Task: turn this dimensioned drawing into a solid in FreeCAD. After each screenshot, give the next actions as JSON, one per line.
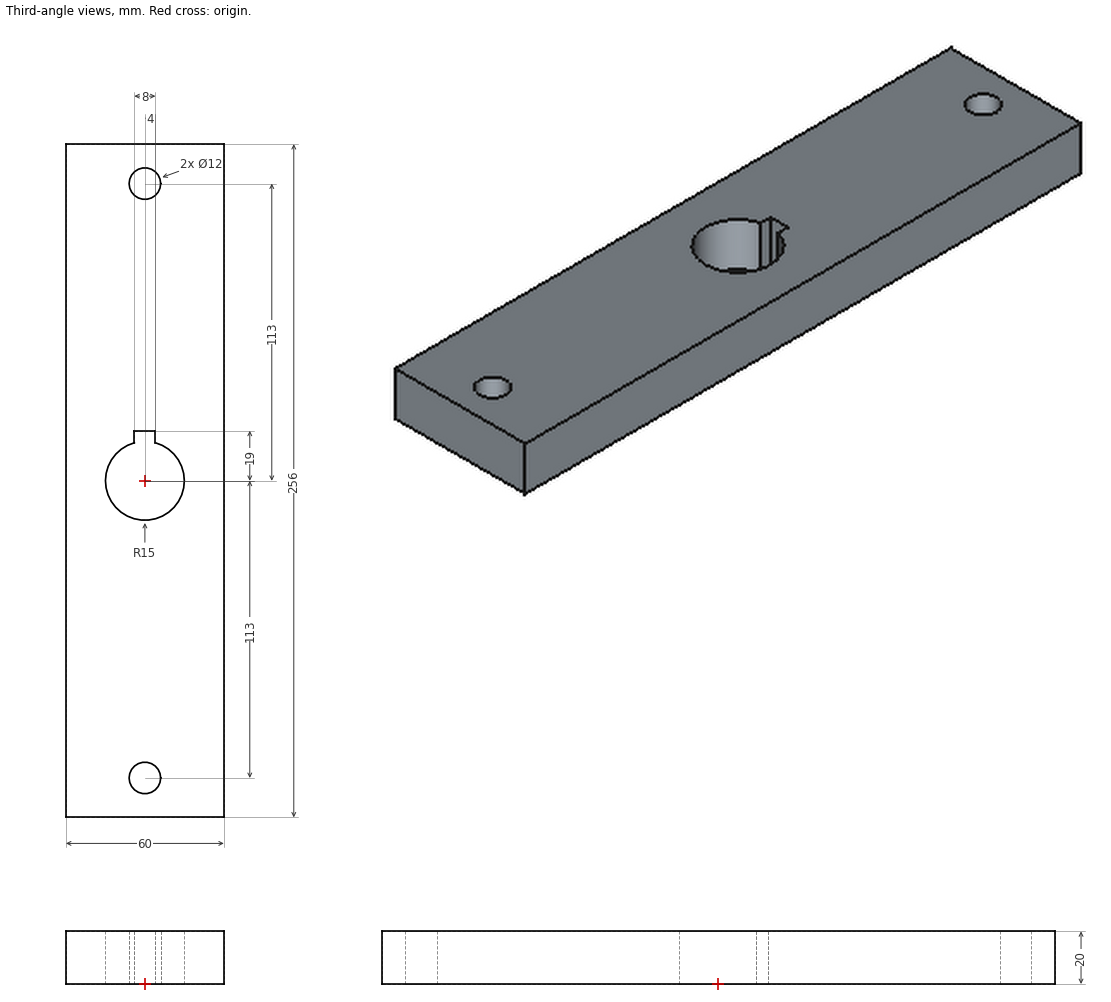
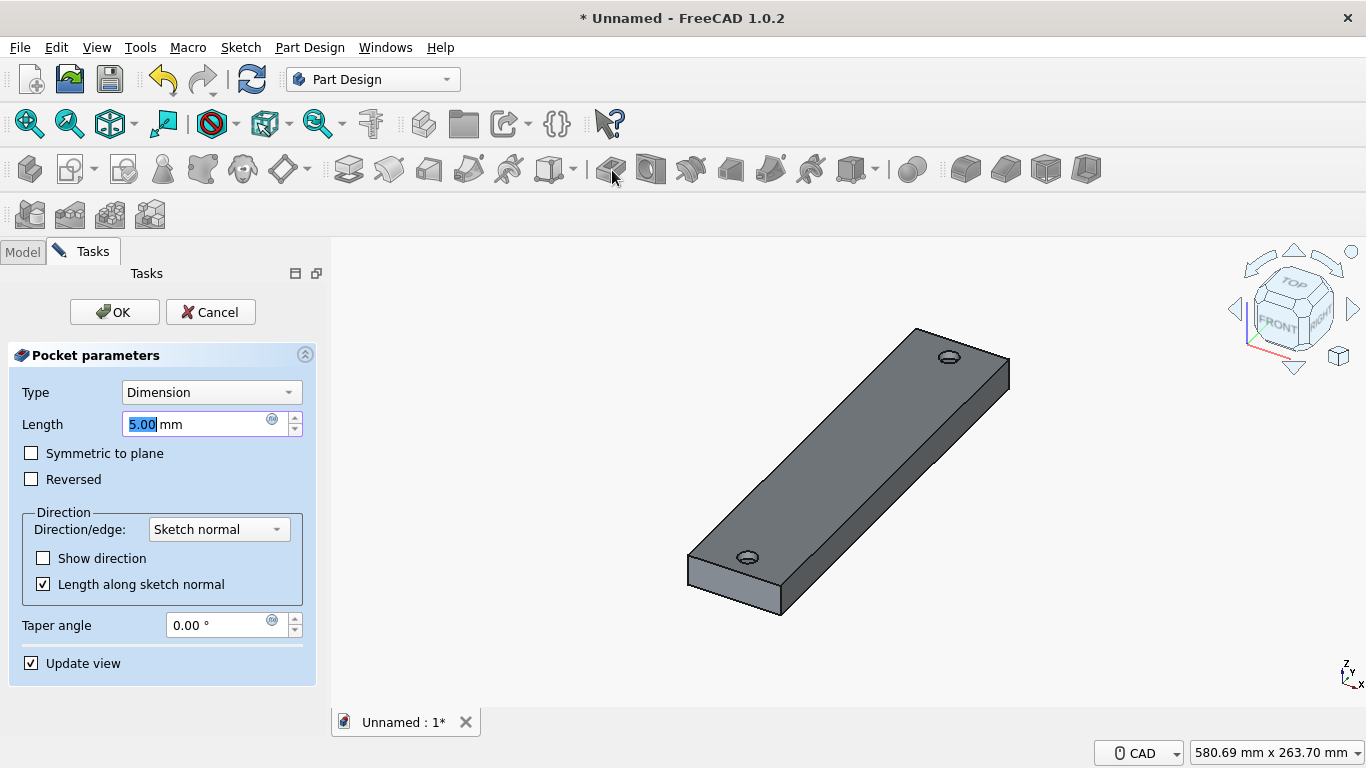
{"action": "left_click", "coordinate": [212, 392]}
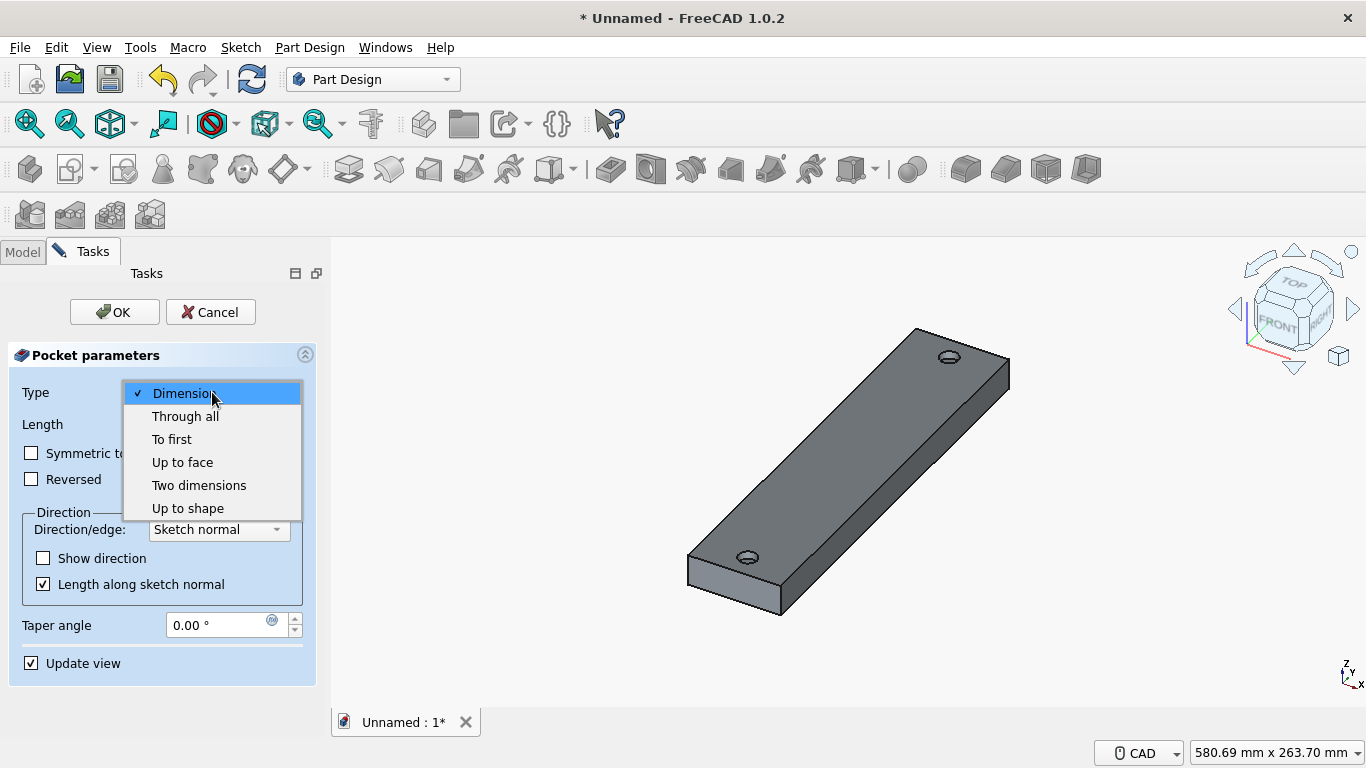
{"action": "left_click", "coordinate": [212, 416]}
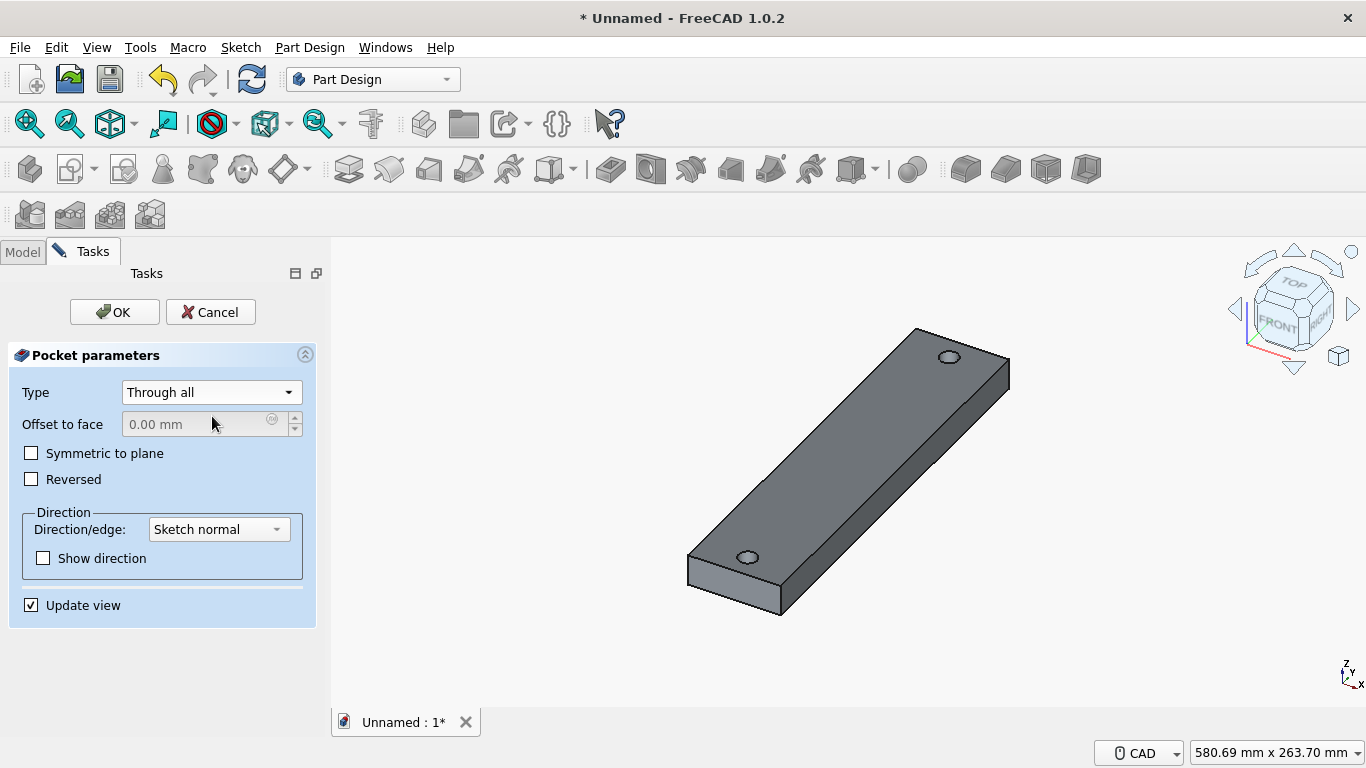
{"action": "left_click", "coordinate": [115, 312]}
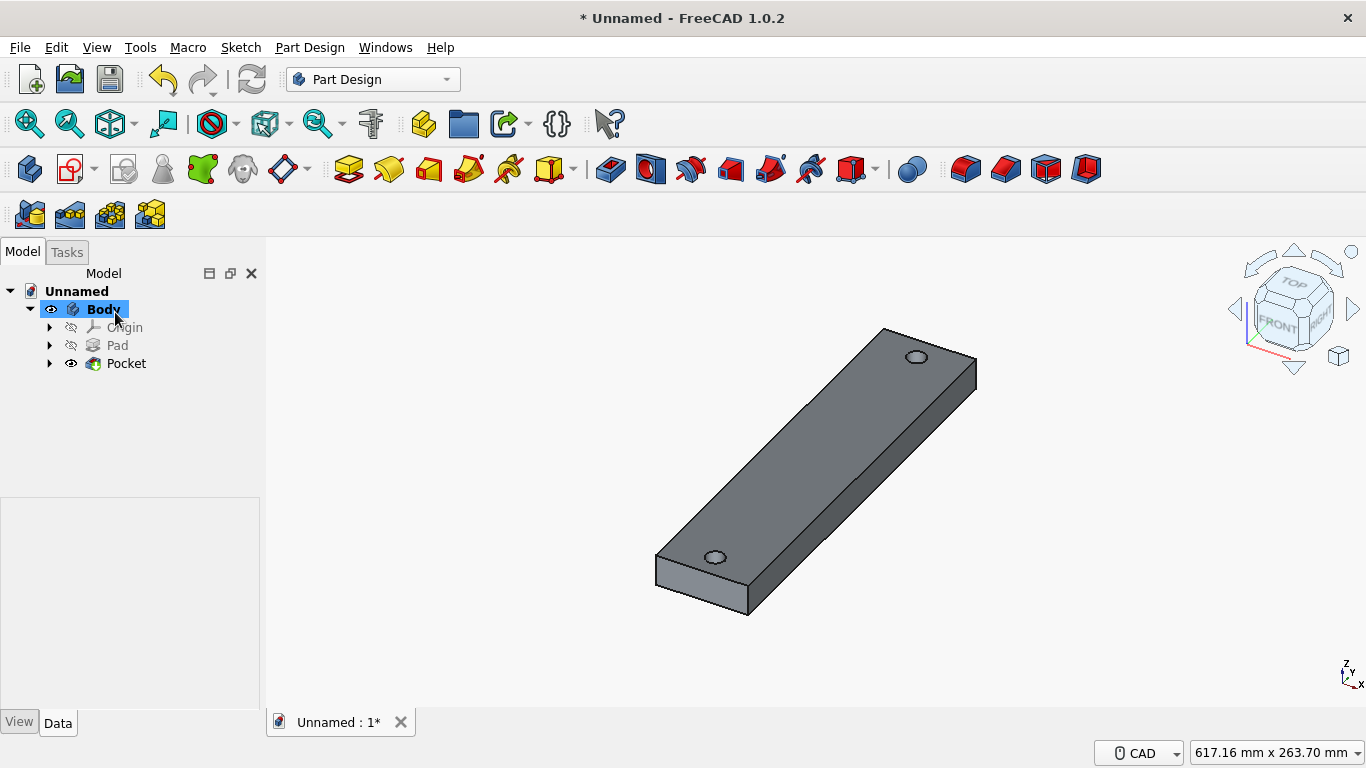
{"action": "left_click", "coordinate": [881, 392]}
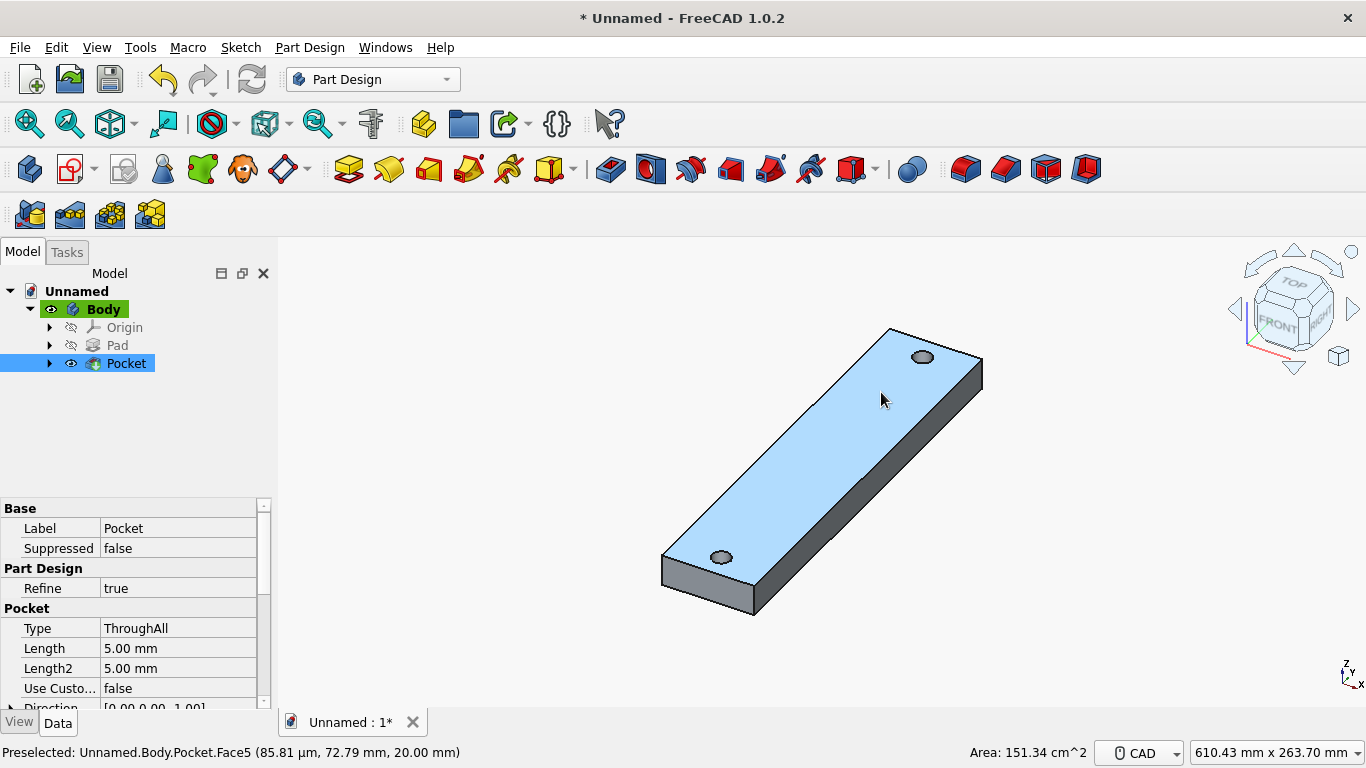
{"action": "left_click", "coordinate": [70, 170]}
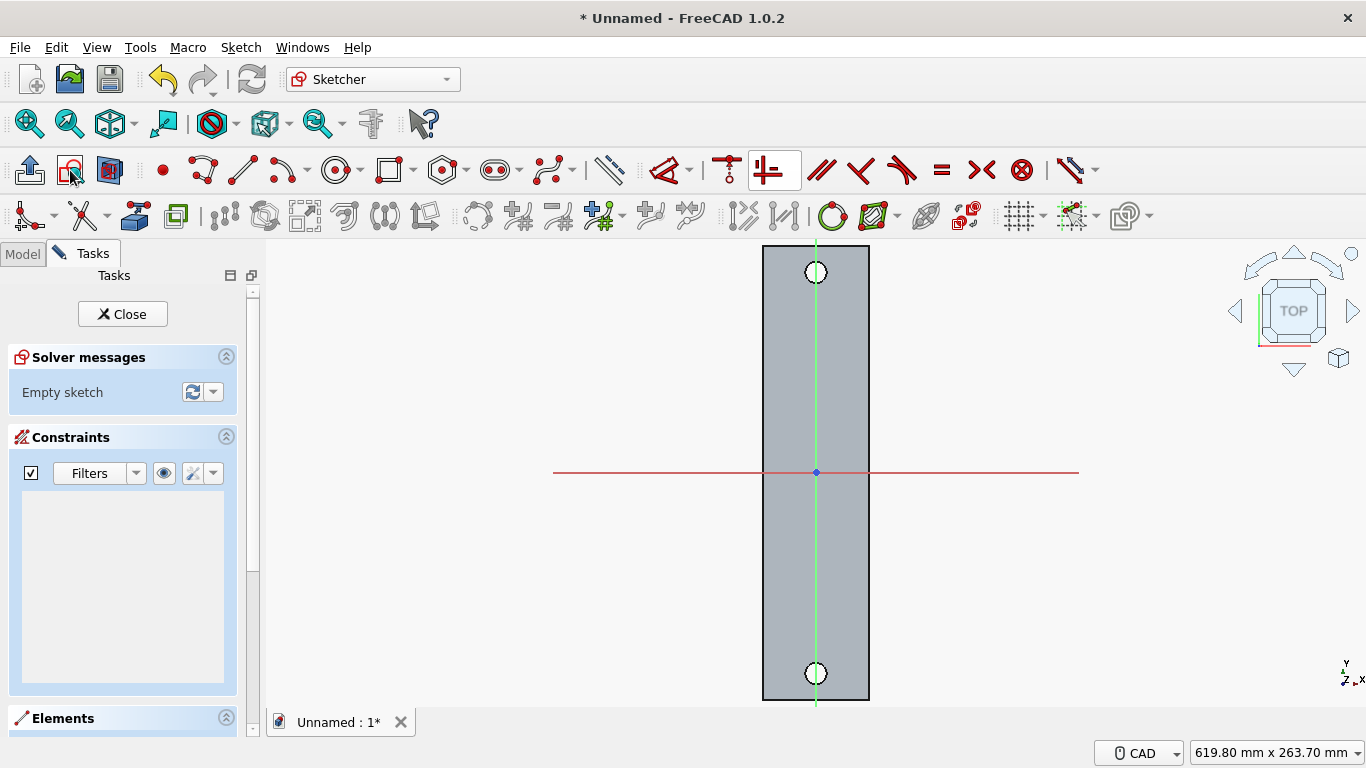
{"action": "scroll", "coordinate": [833, 469], "scroll_direction": "up", "scroll_amount": 8}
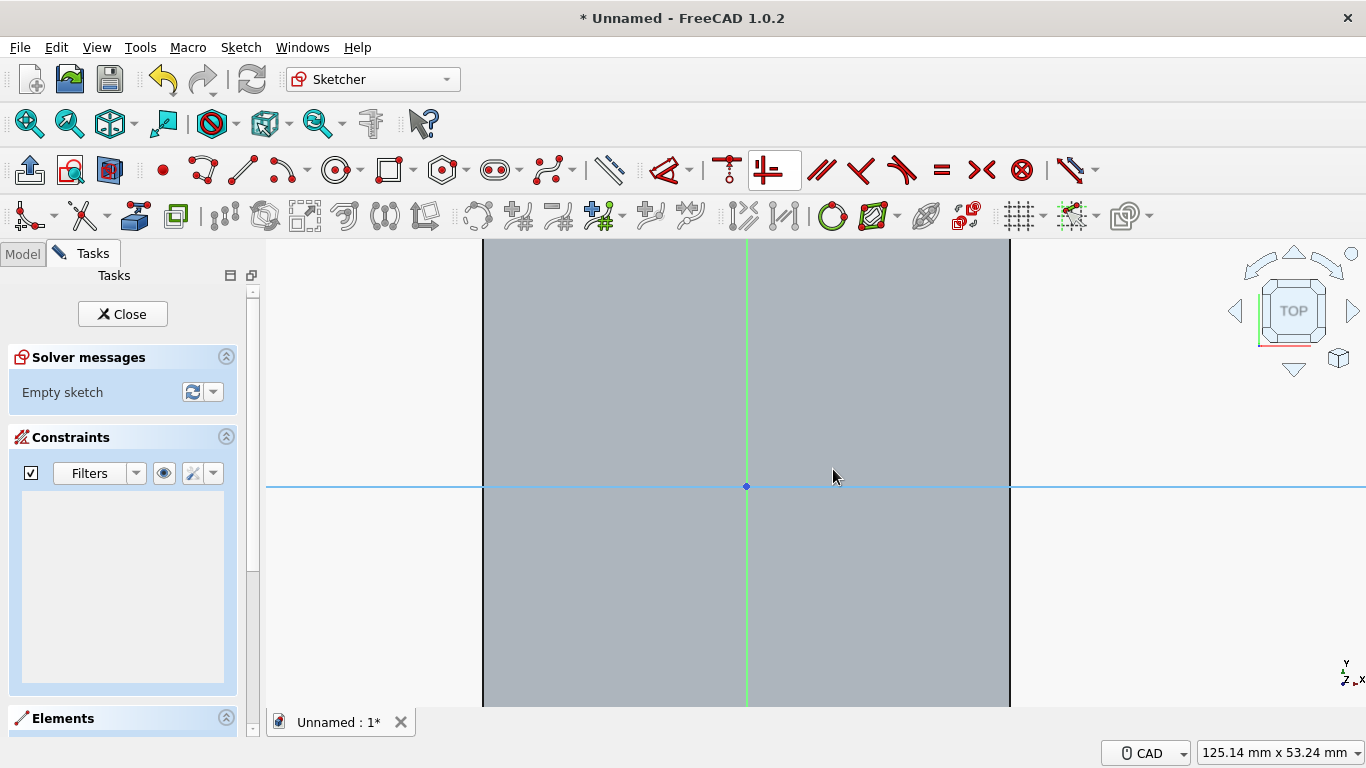
{"action": "key", "text": "g m"}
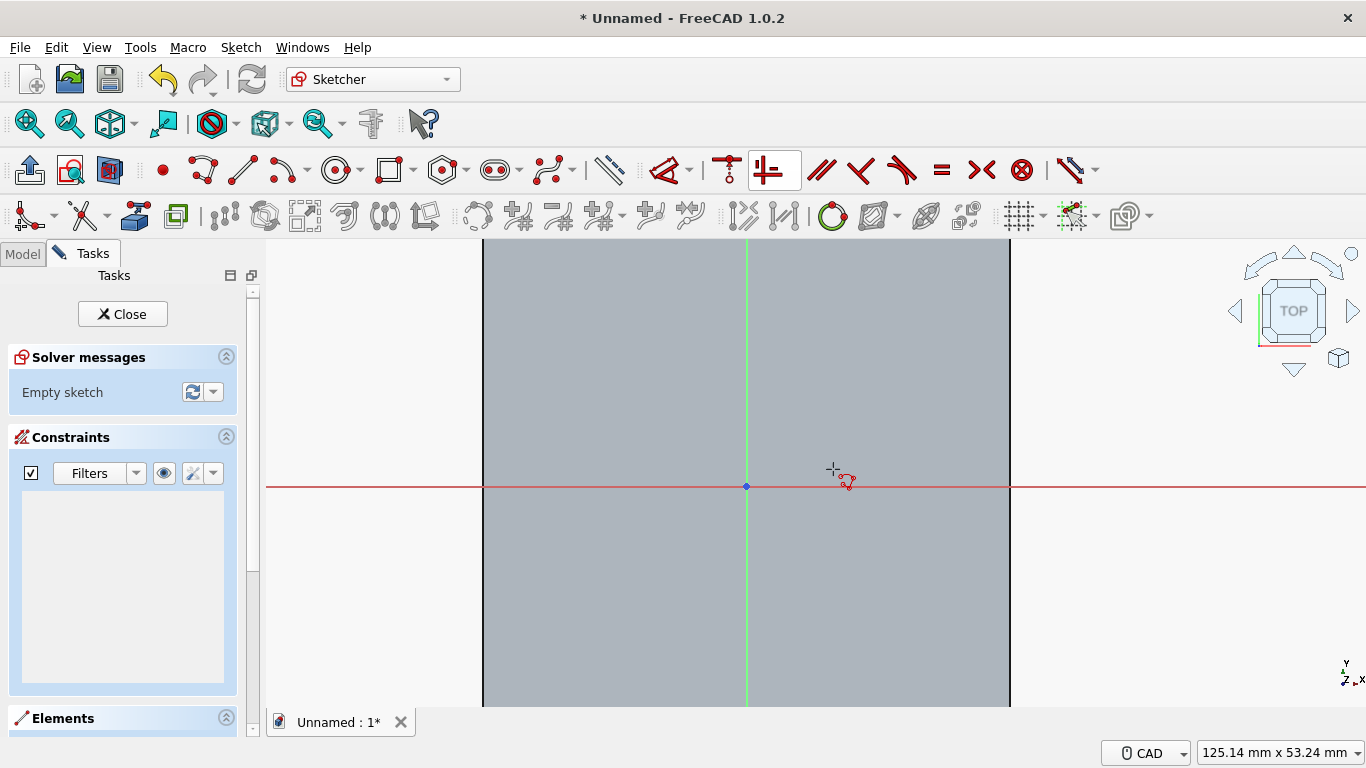
{"action": "left_click", "coordinate": [782, 360]}
{"action": "left_click", "coordinate": [782, 320]}
{"action": "left_click", "coordinate": [712, 320]}
{"action": "left_click", "coordinate": [712, 360]}
{"action": "right_click", "coordinate": [712, 360]}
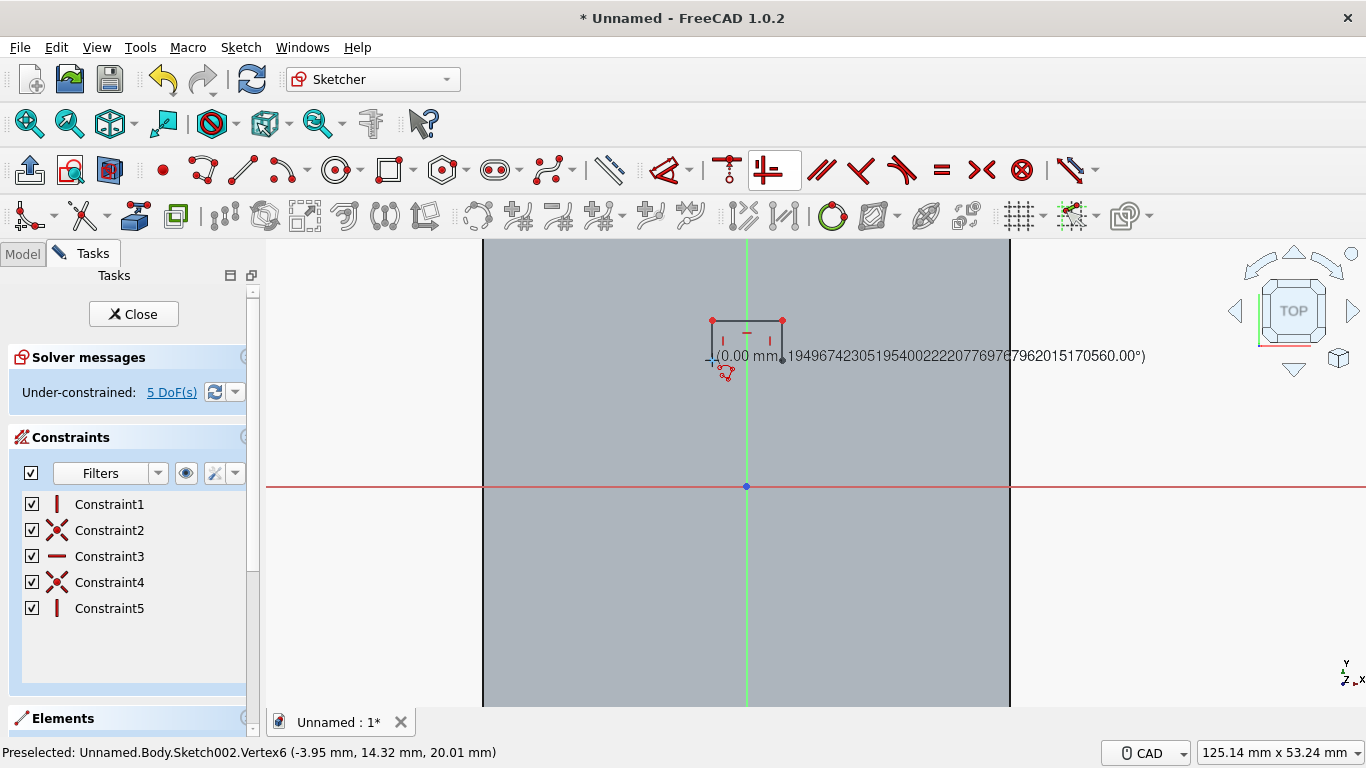
{"action": "key", "text": "g 3 a"}